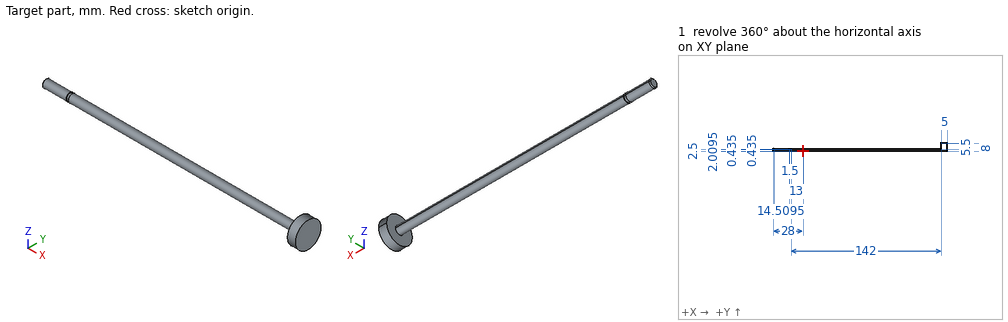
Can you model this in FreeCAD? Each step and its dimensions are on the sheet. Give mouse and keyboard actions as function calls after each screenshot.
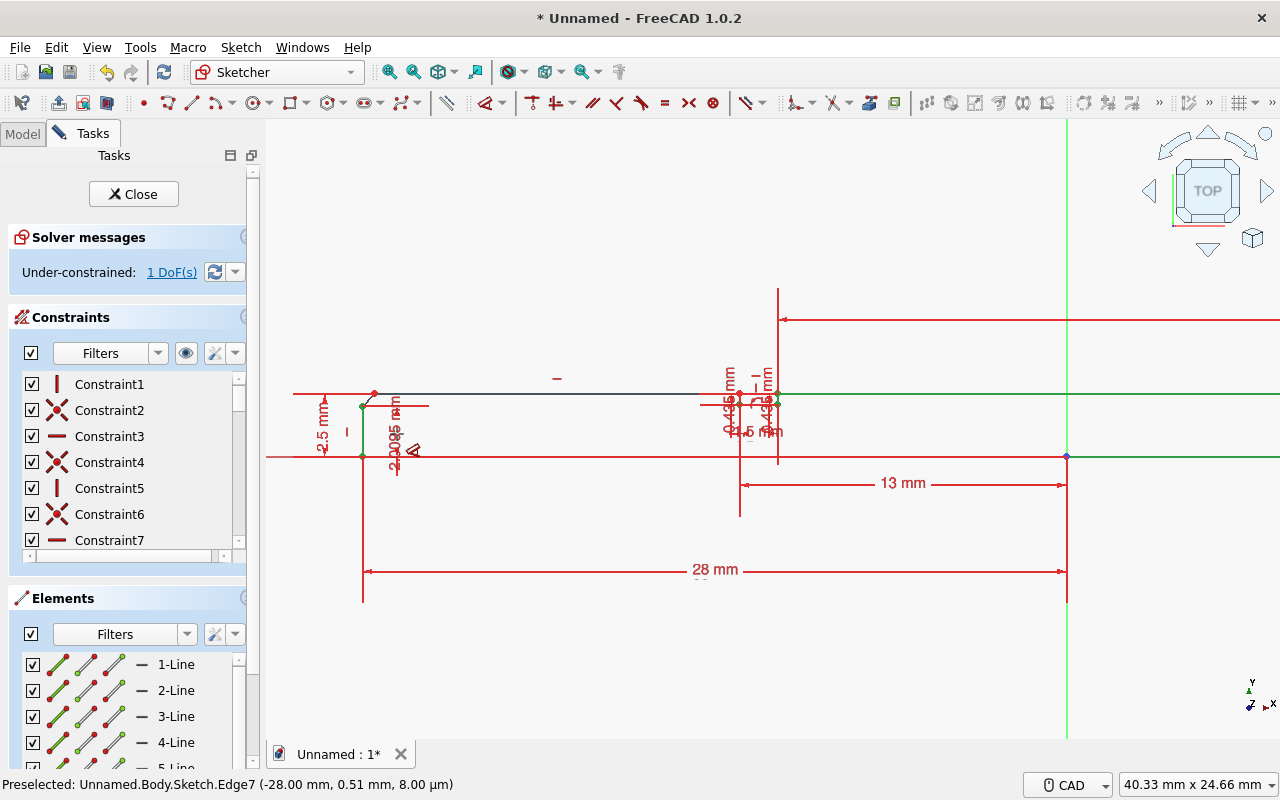
scroll(436, 440, down, 10)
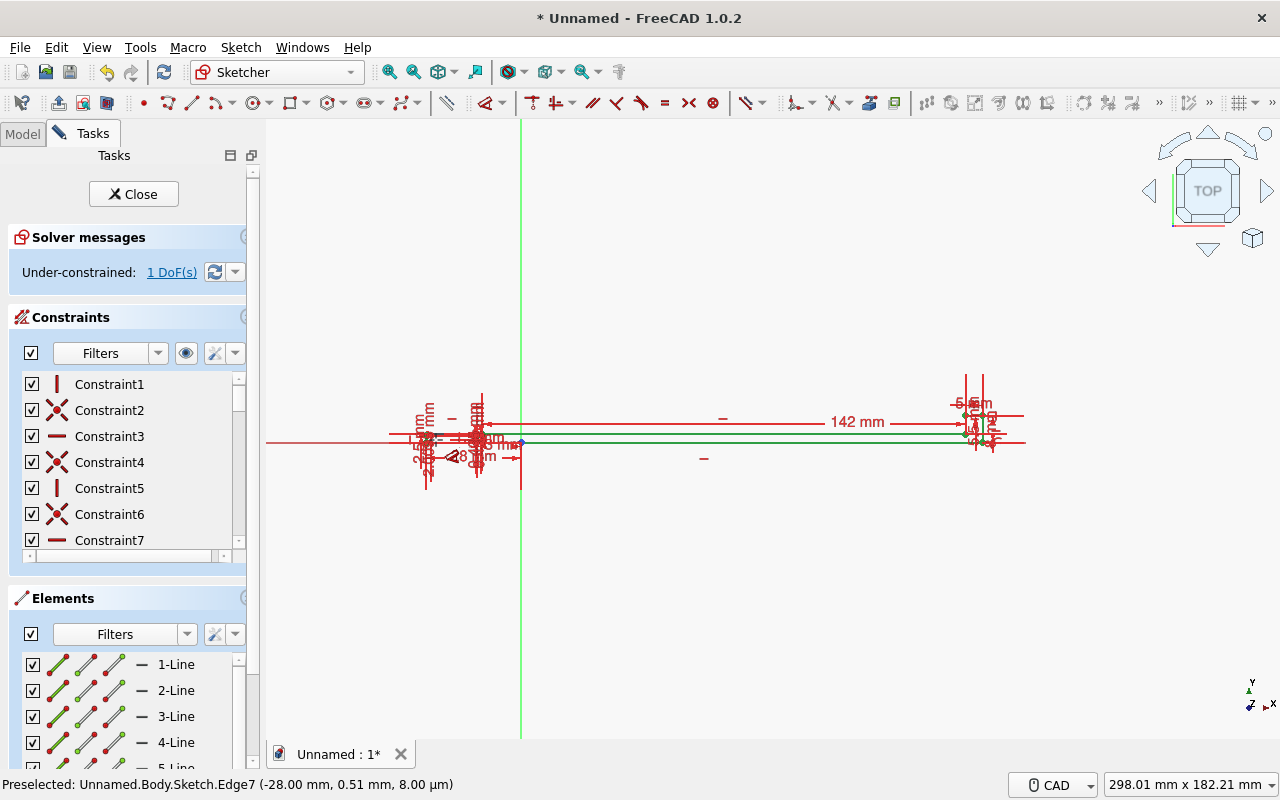
scroll(443, 434, up, 3)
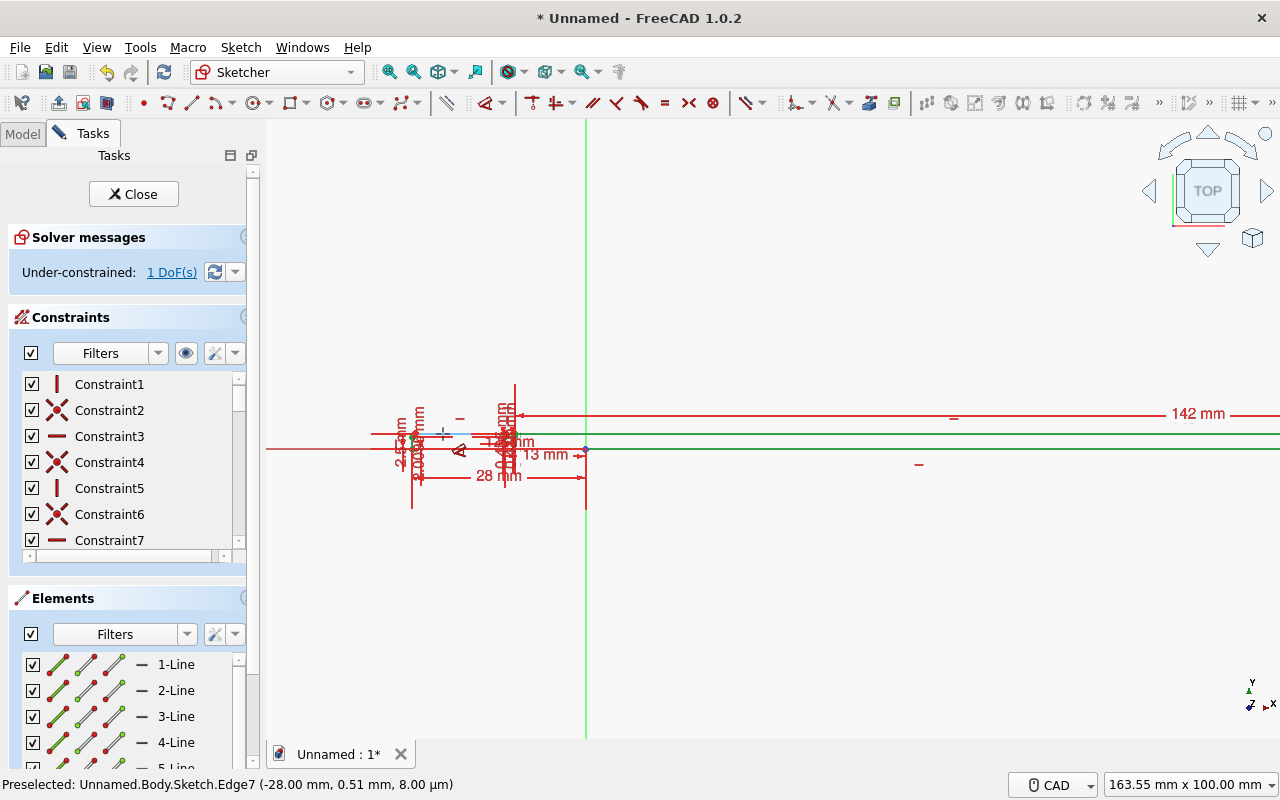
click(442, 434)
click(429, 468)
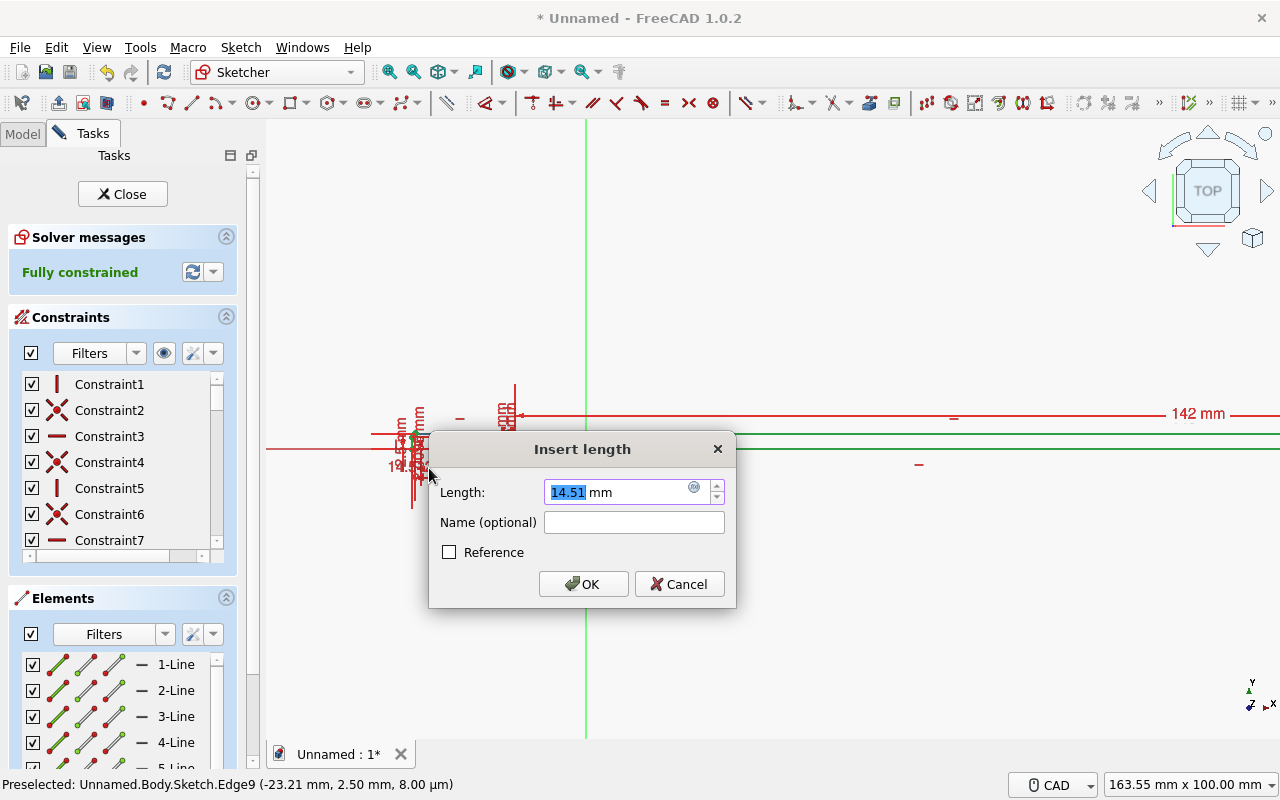
text(14.5095)
key(Return)
key(Escape)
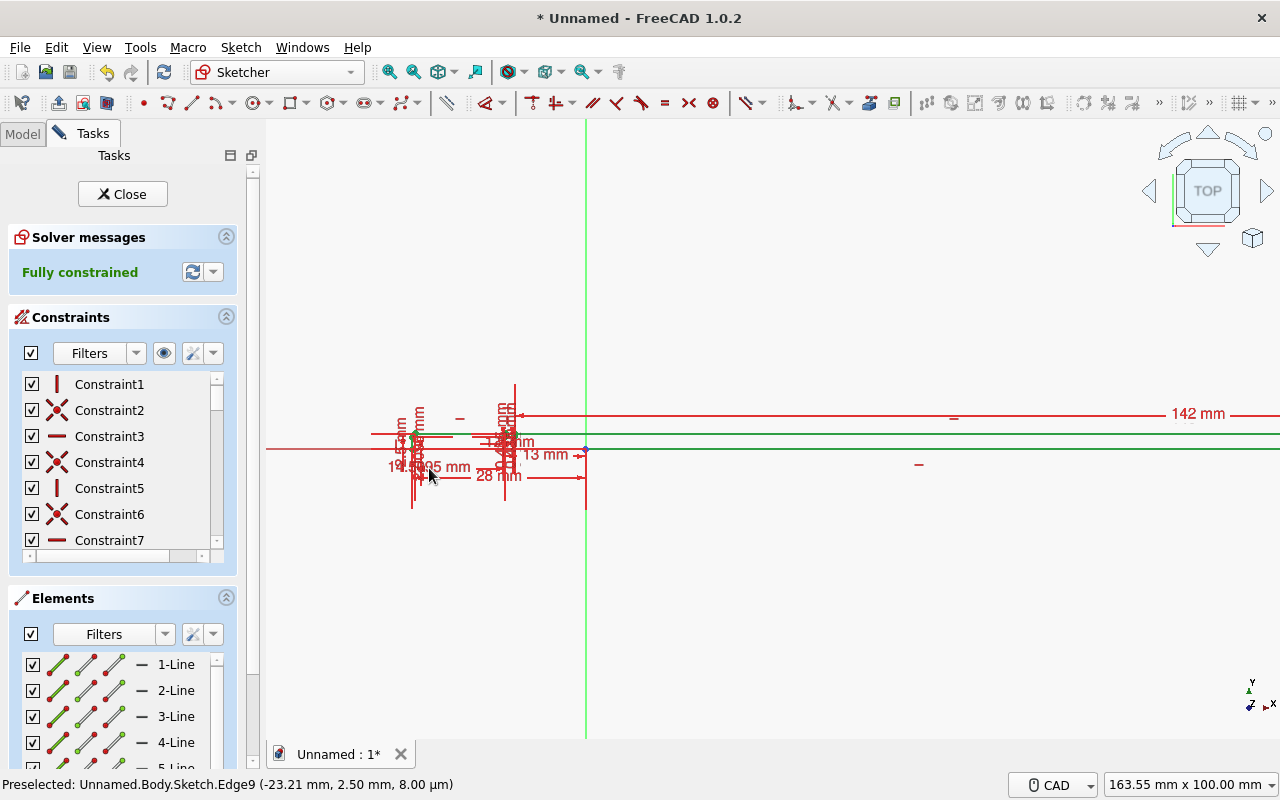
click(123, 194)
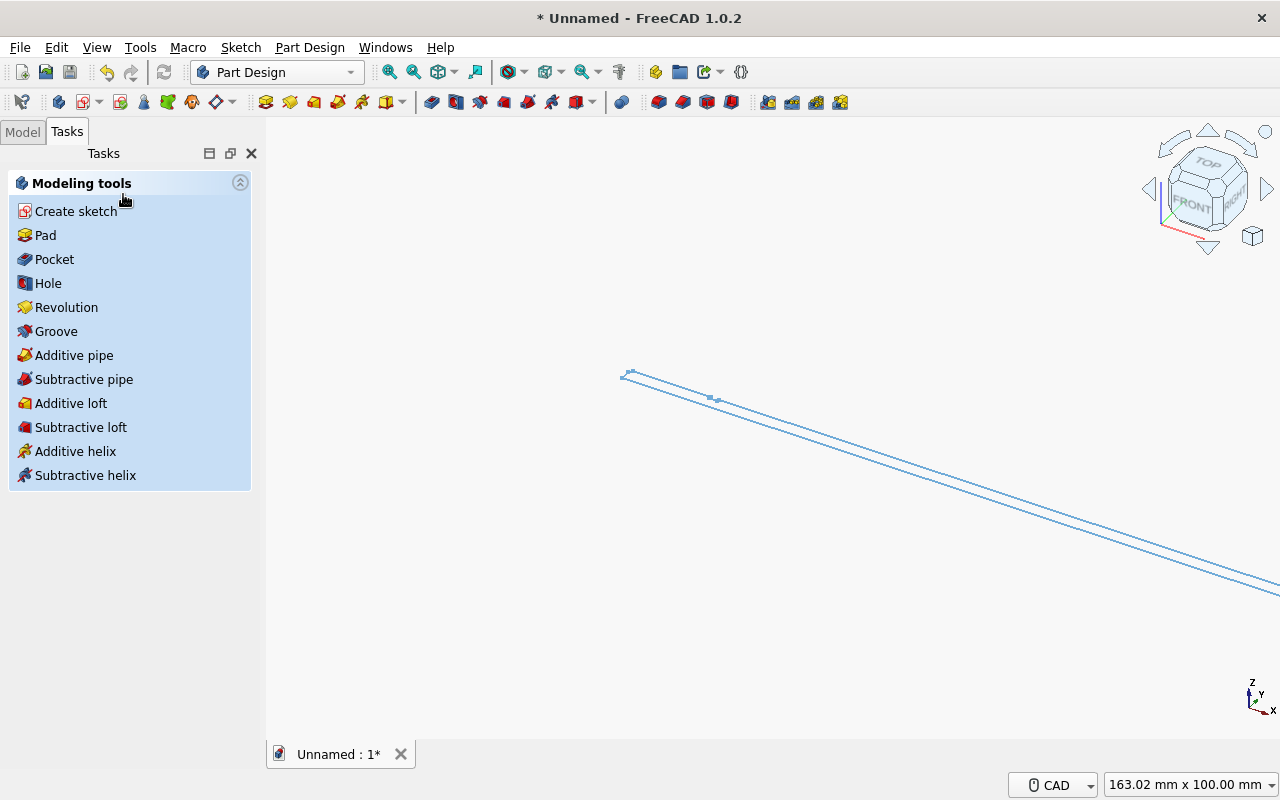
click(290, 102)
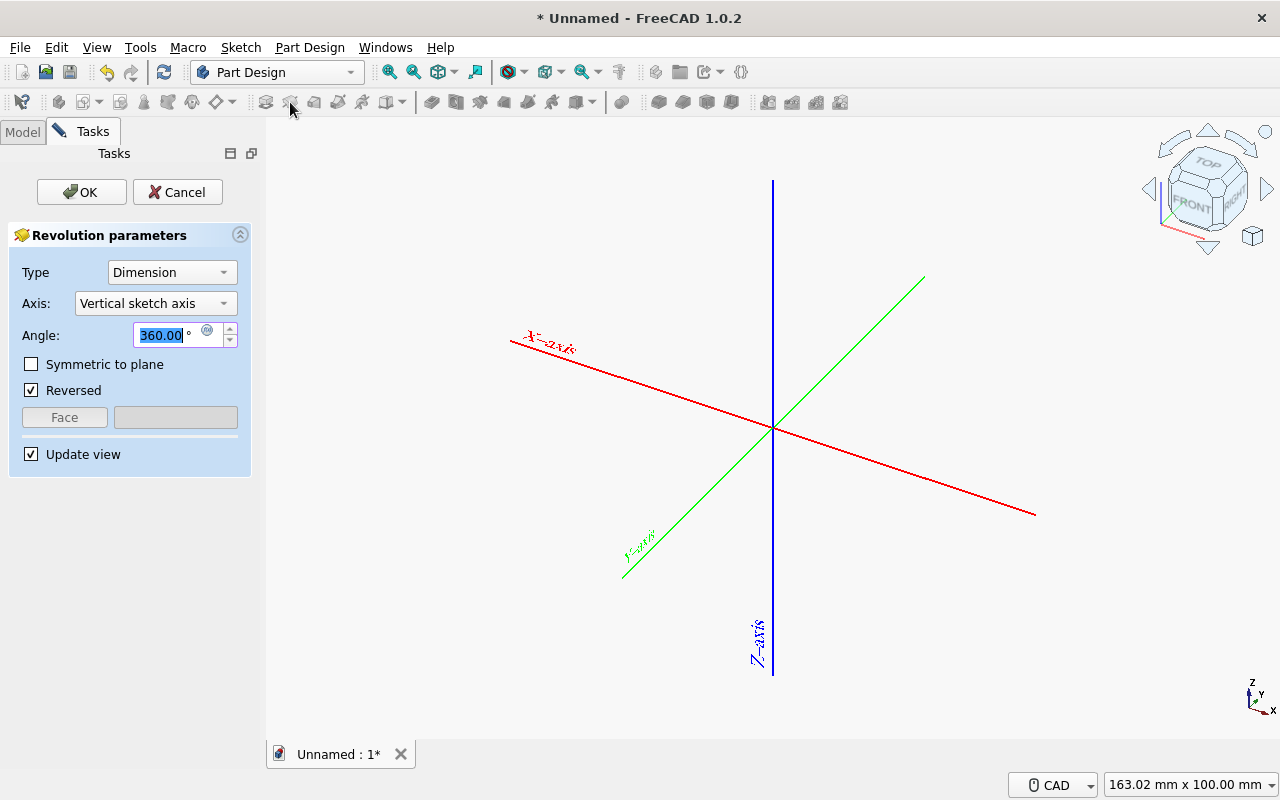
click(156, 304)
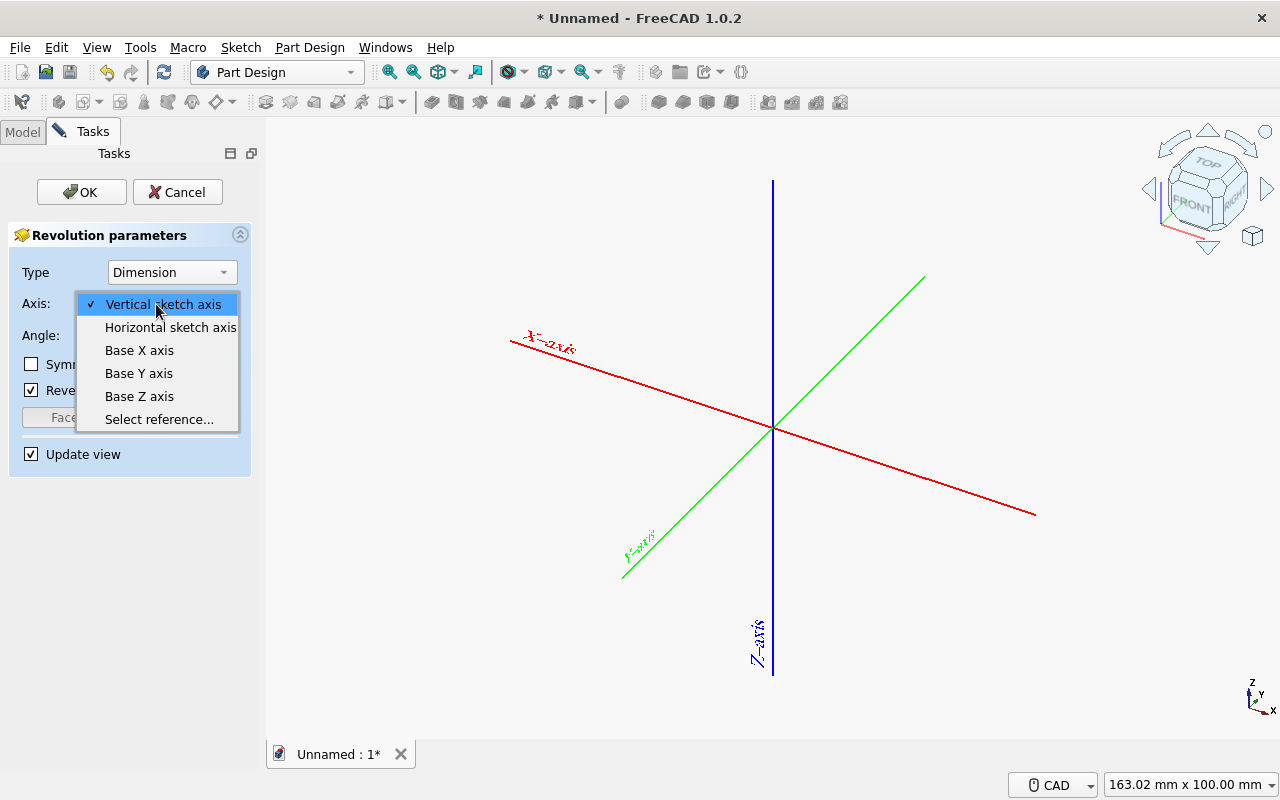
click(156, 328)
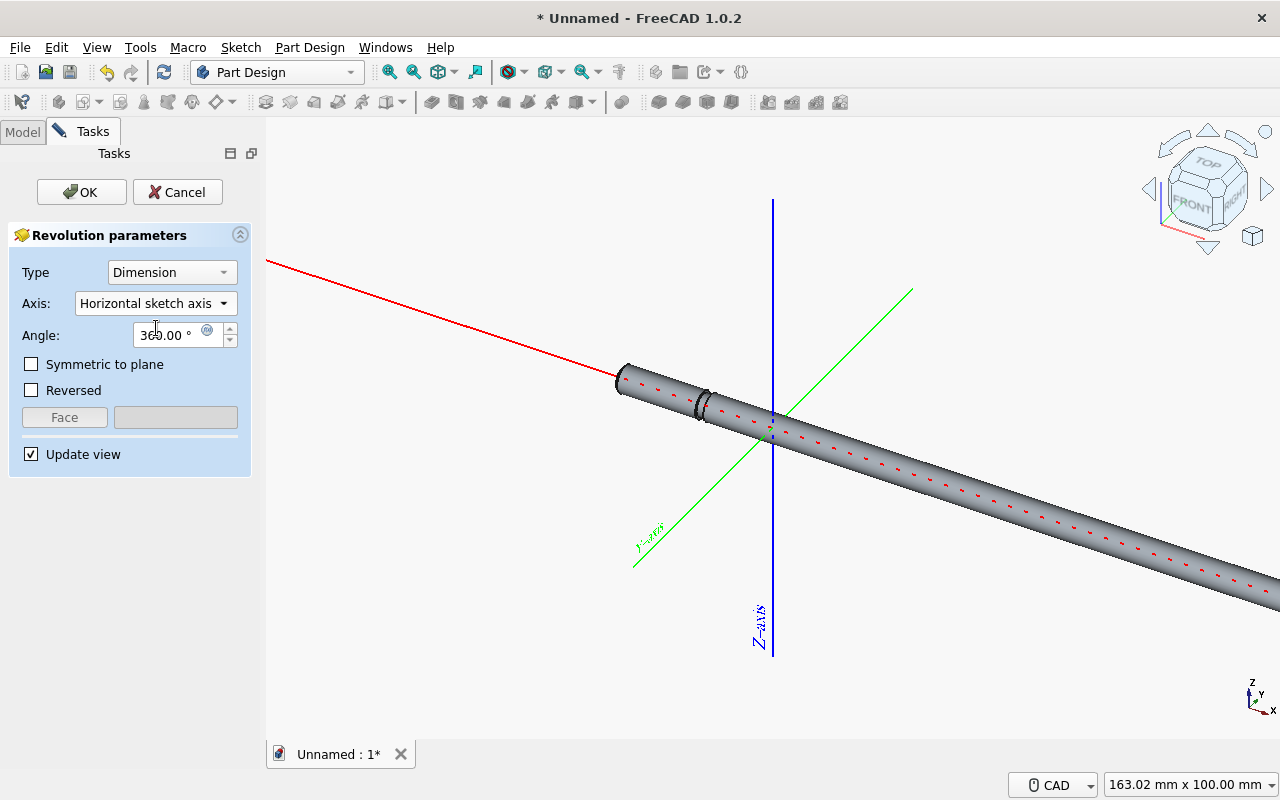
click(82, 192)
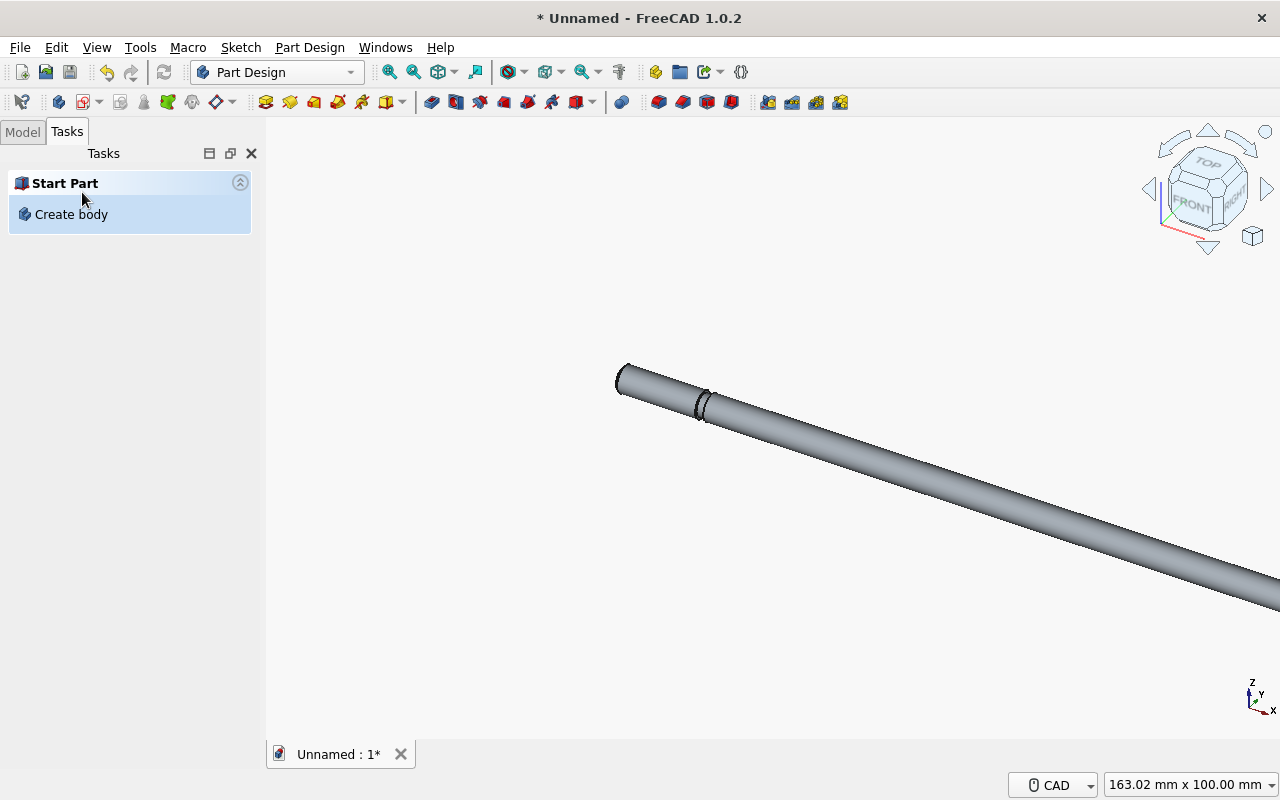
key(0)